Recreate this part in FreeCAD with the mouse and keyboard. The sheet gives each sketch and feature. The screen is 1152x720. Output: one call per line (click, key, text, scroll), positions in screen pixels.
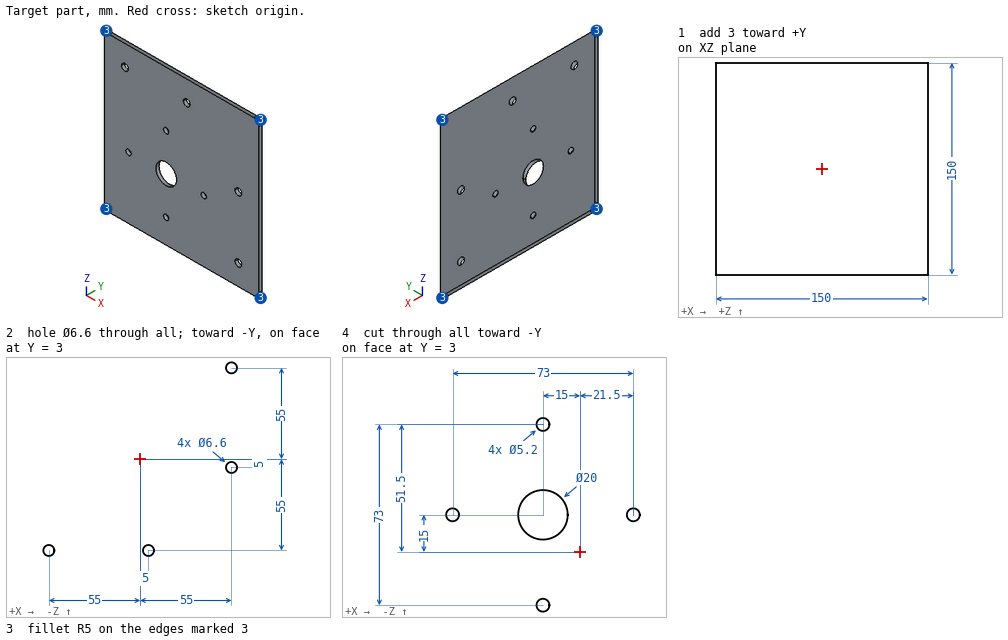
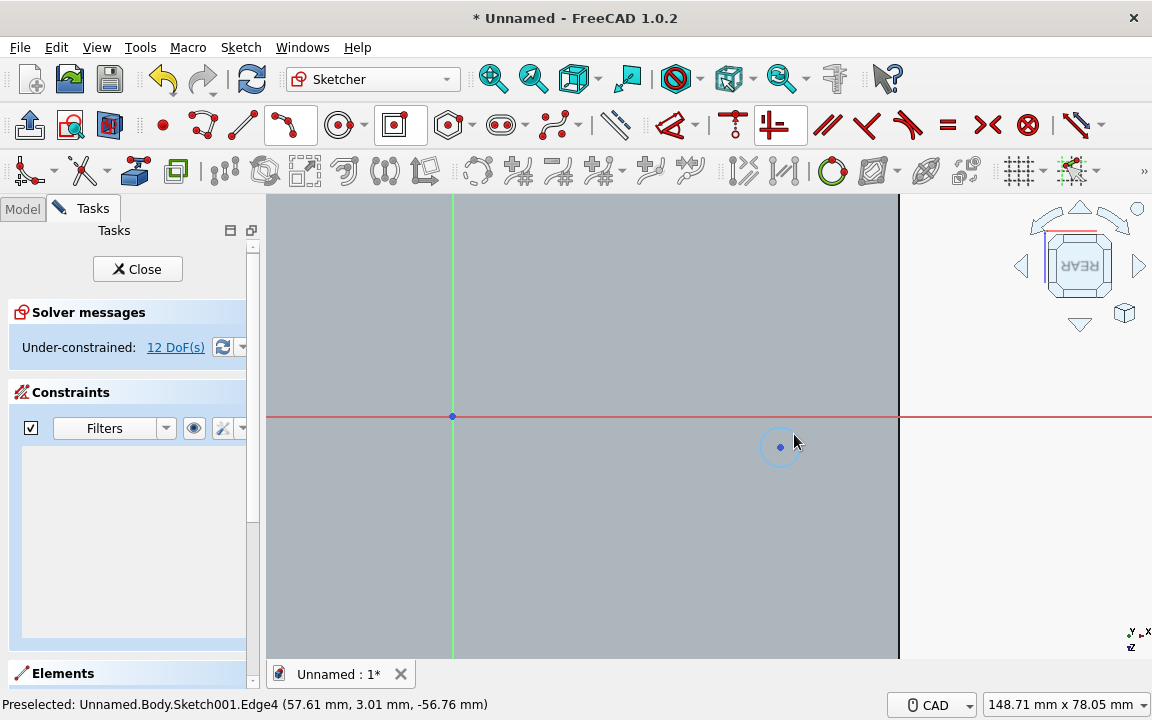
click(794, 433)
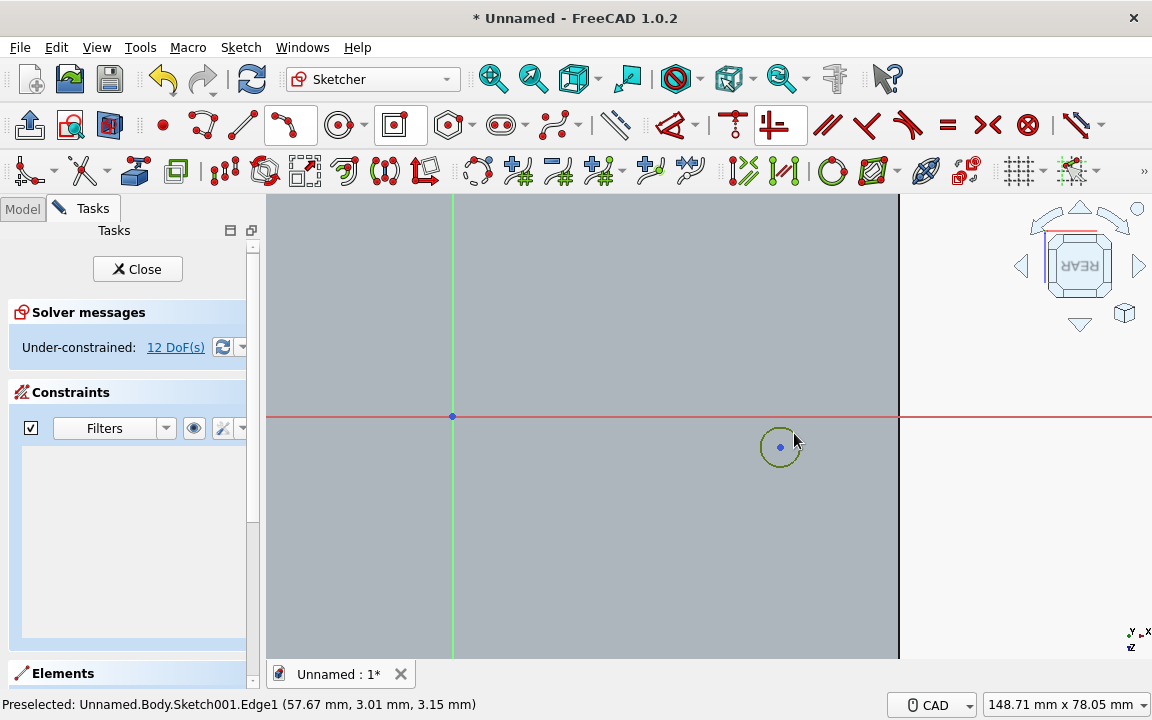
scroll(794, 434, down, 4)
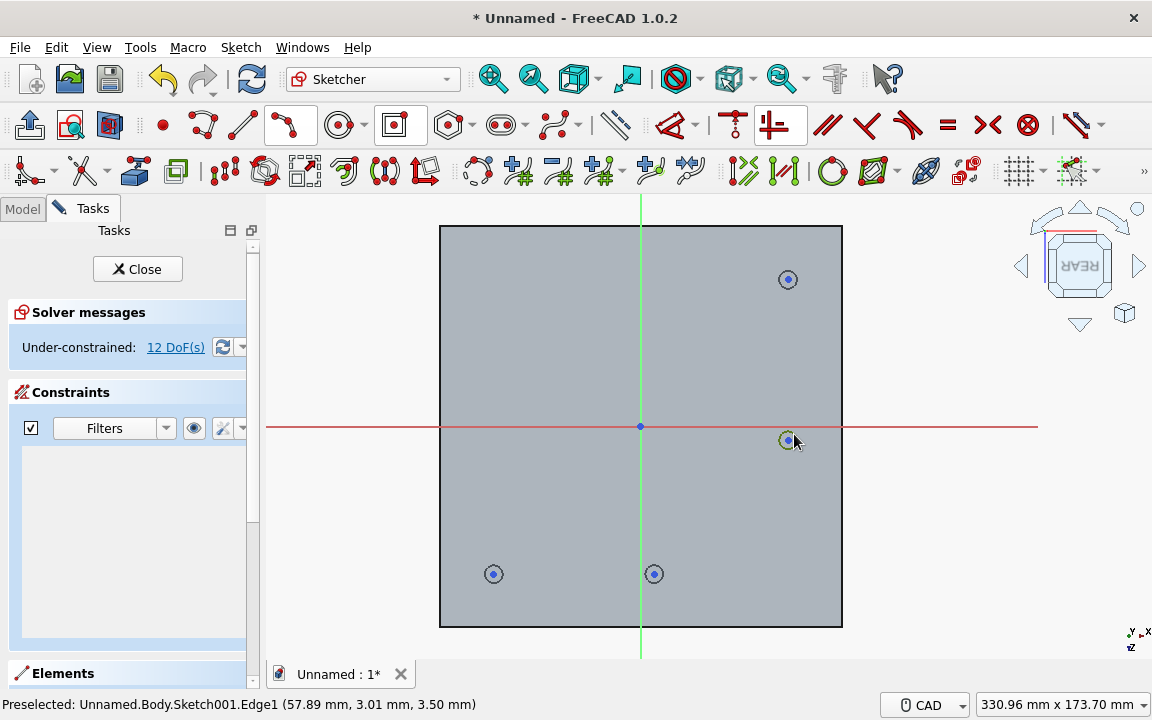
scroll(661, 568, up, 3)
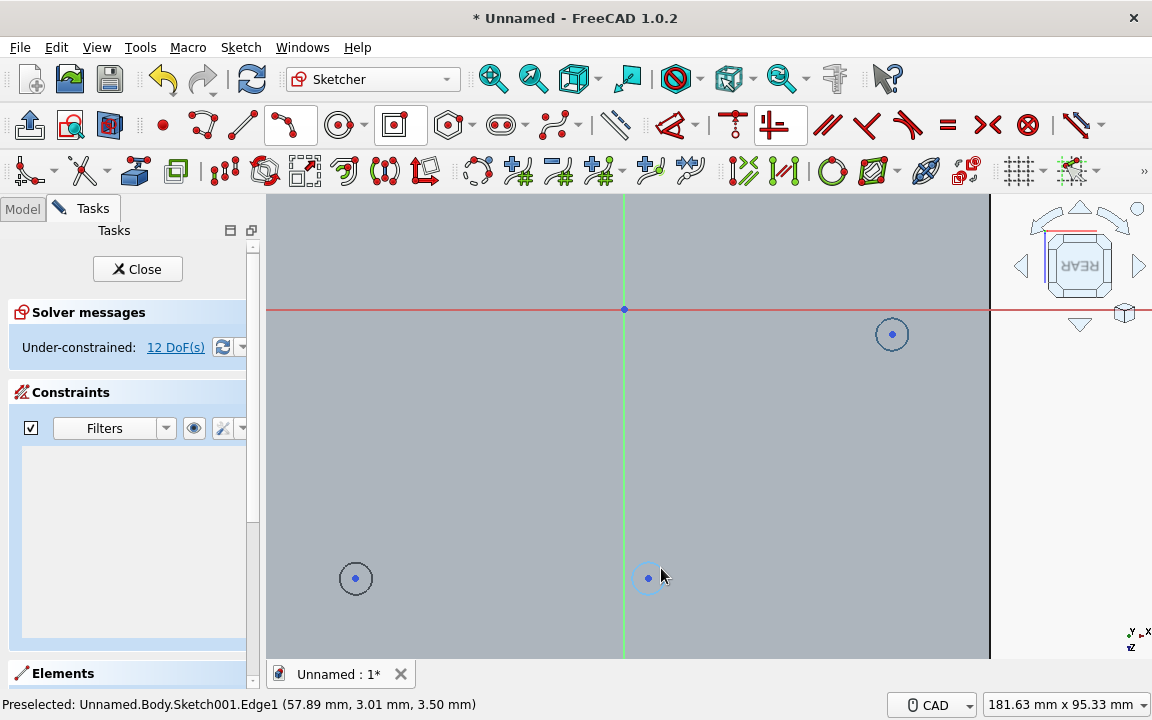
click(660, 567)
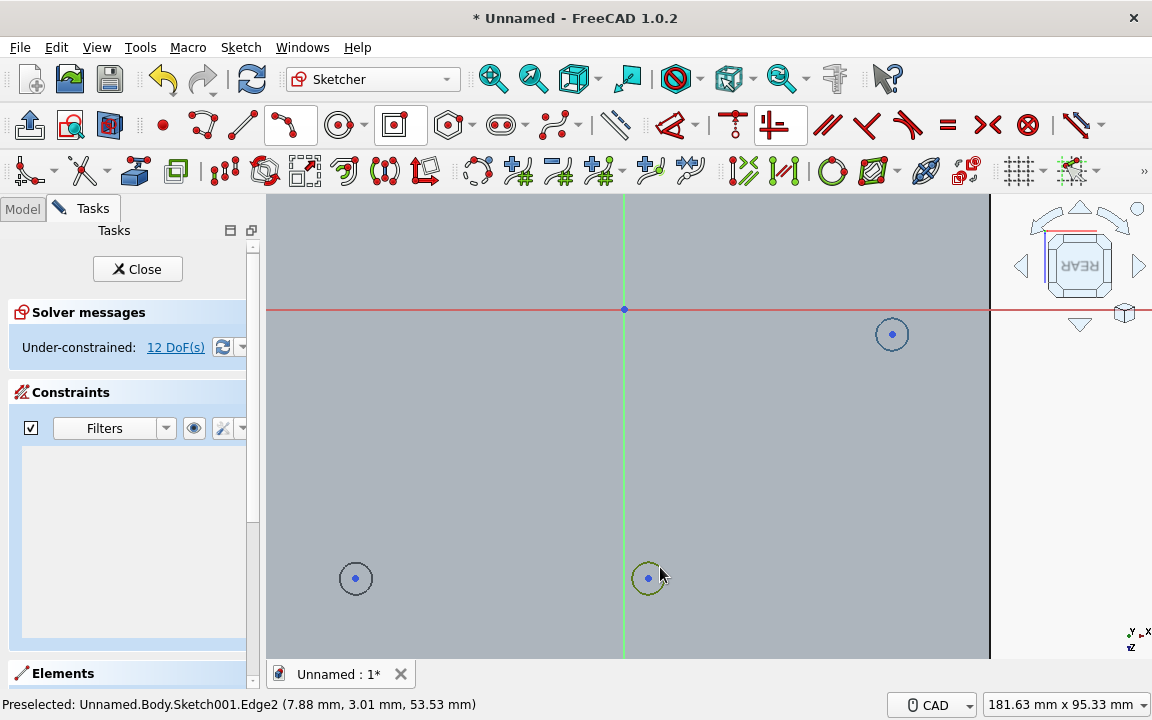
click(367, 567)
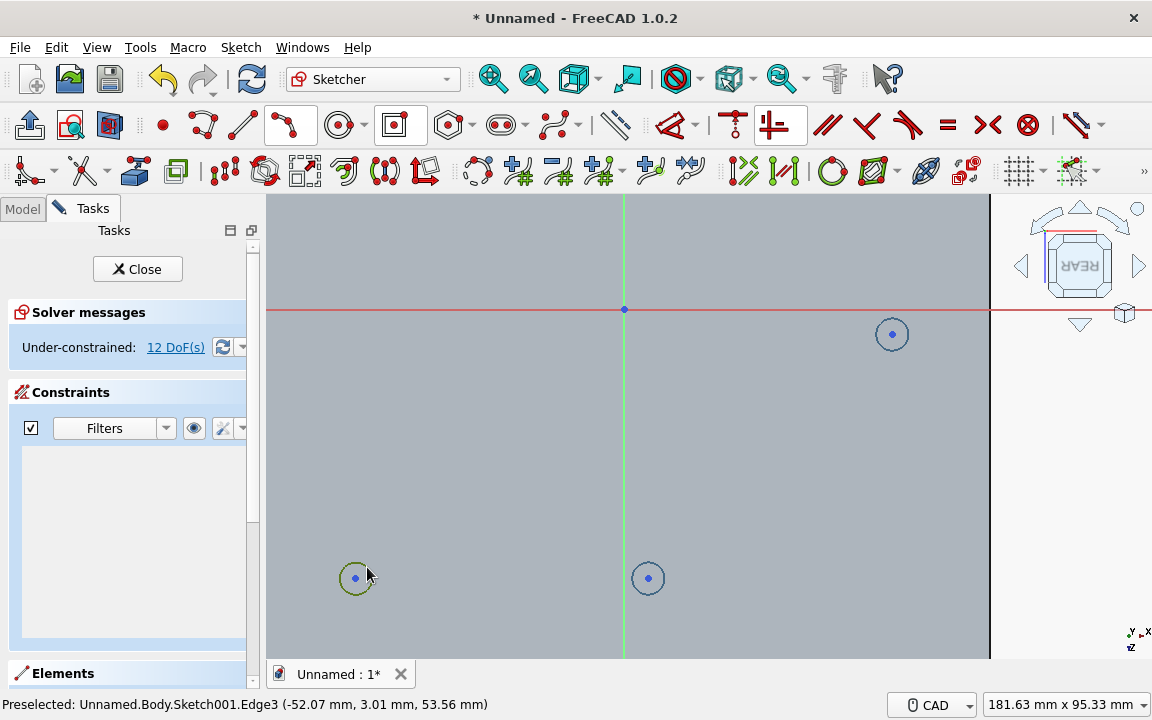
scroll(660, 569, down, 3)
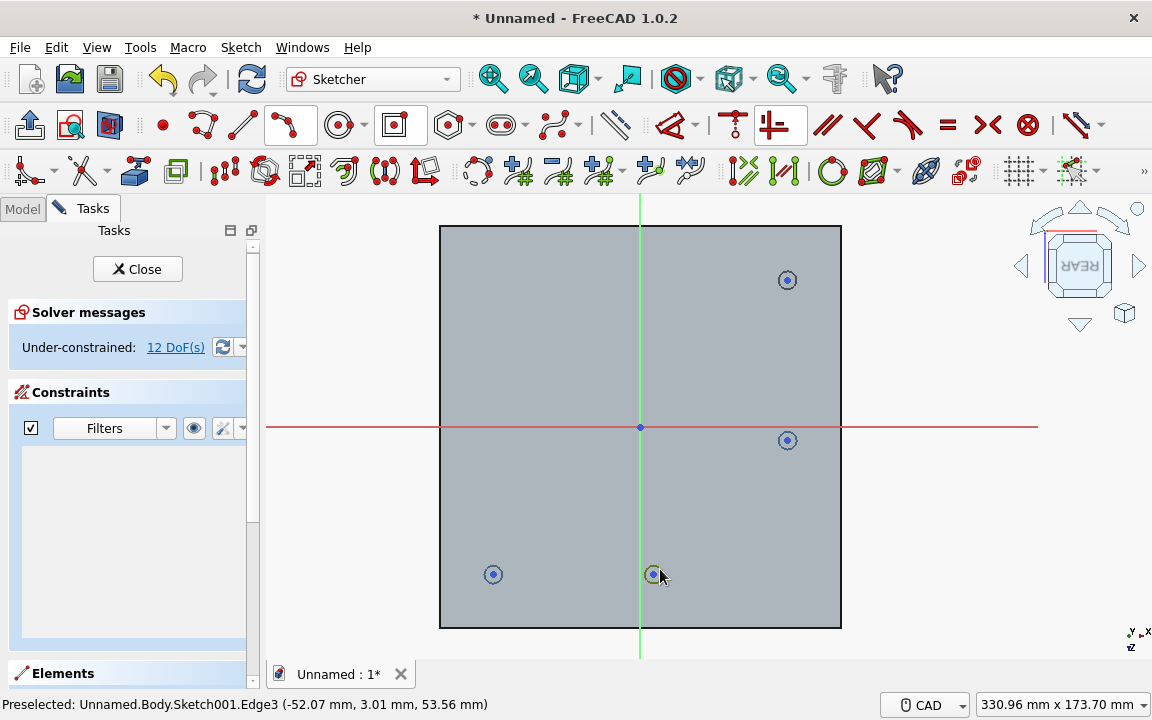
scroll(794, 274, up, 3)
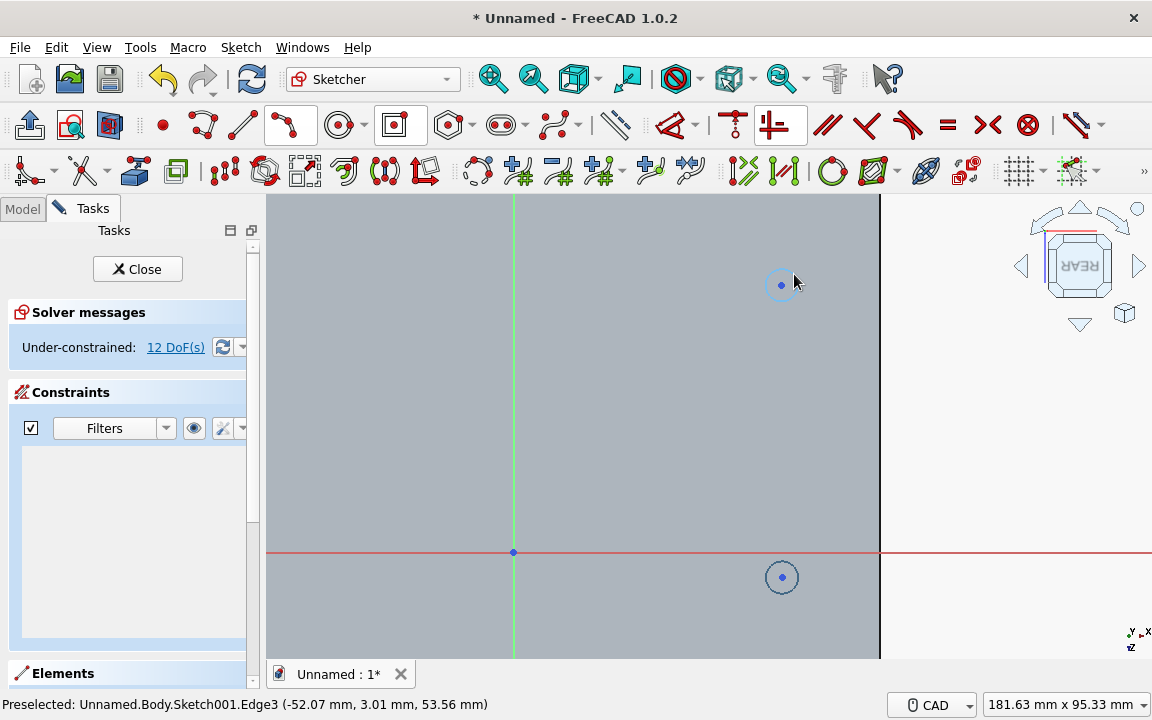
click(793, 274)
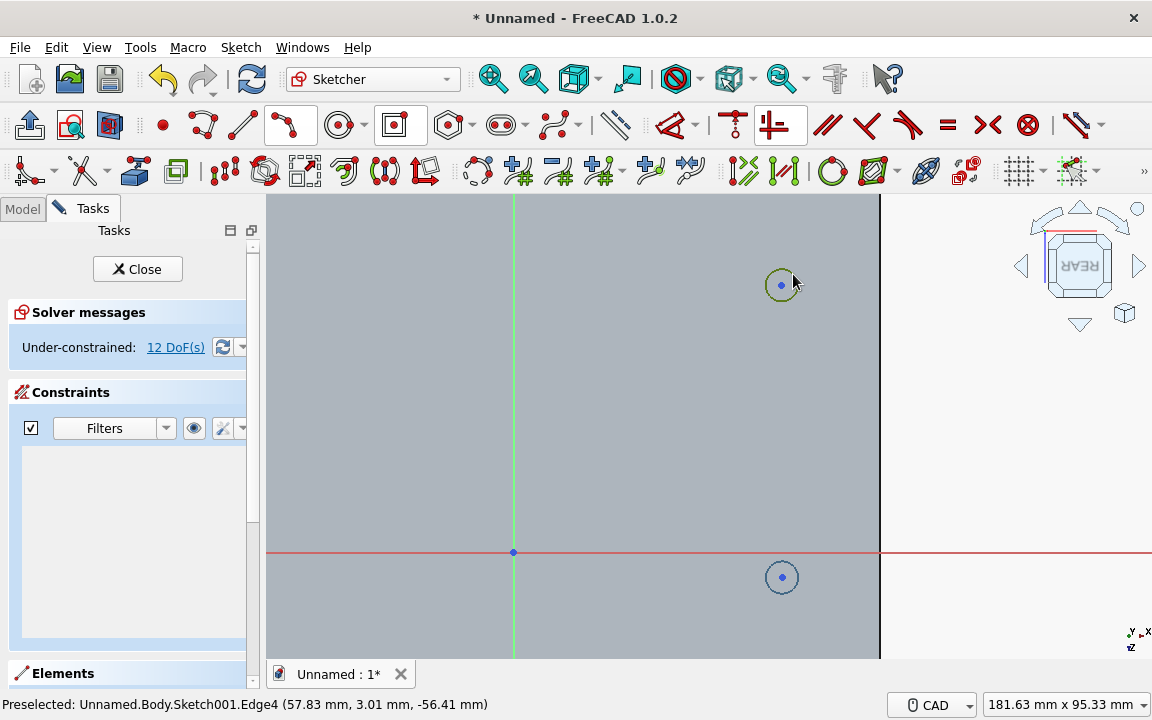
click(948, 126)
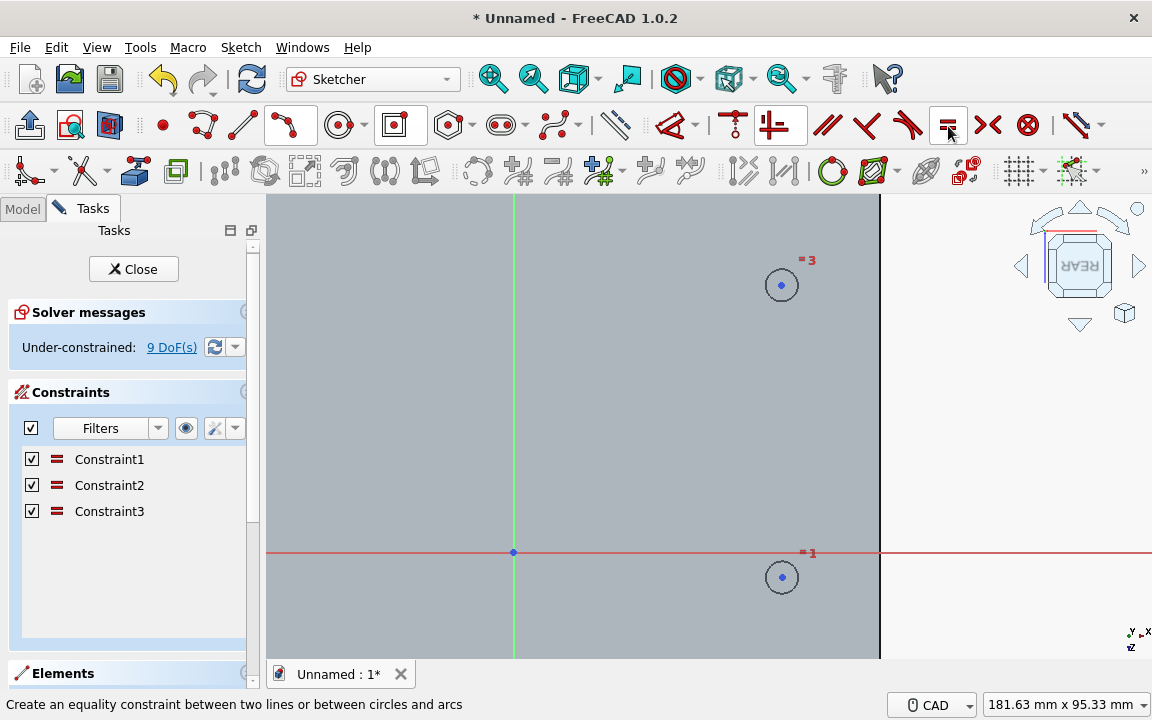
scroll(795, 273, down, 3)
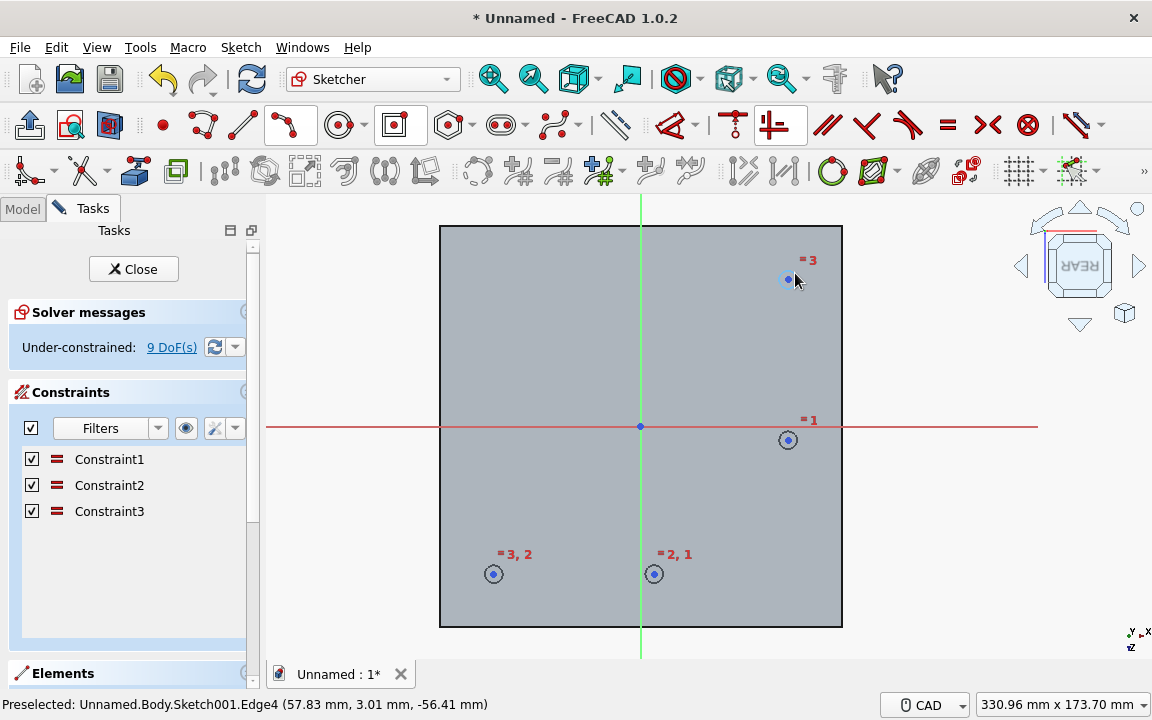
click(654, 574)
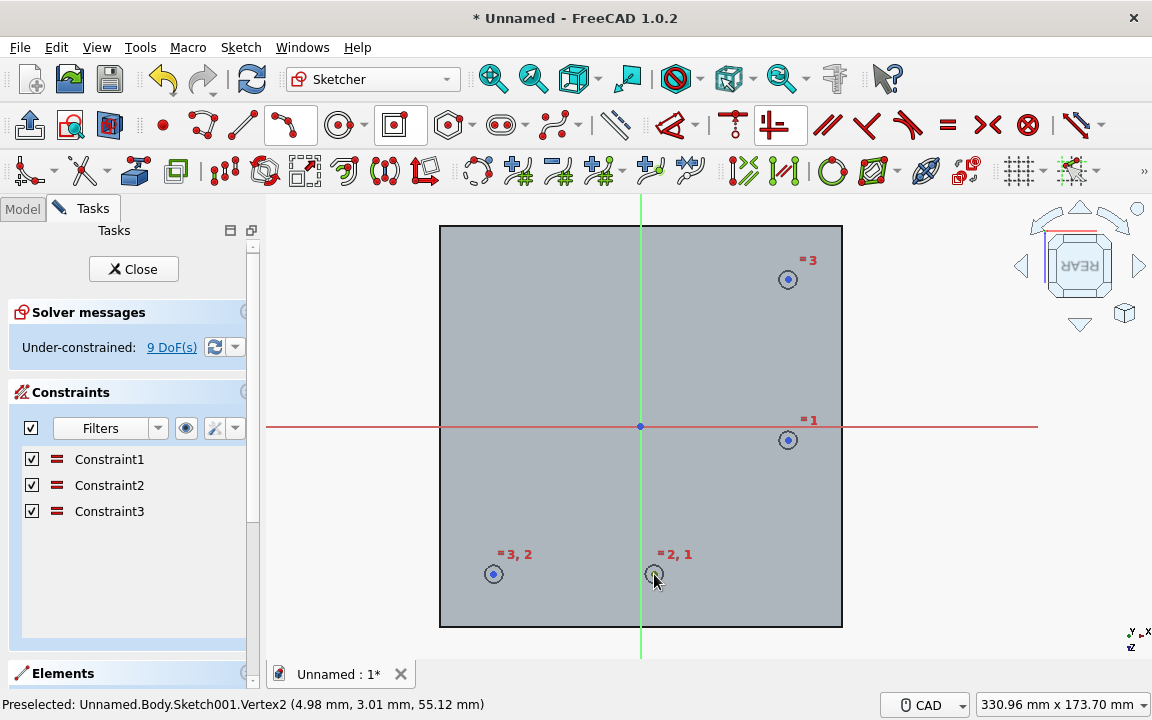
click(494, 574)